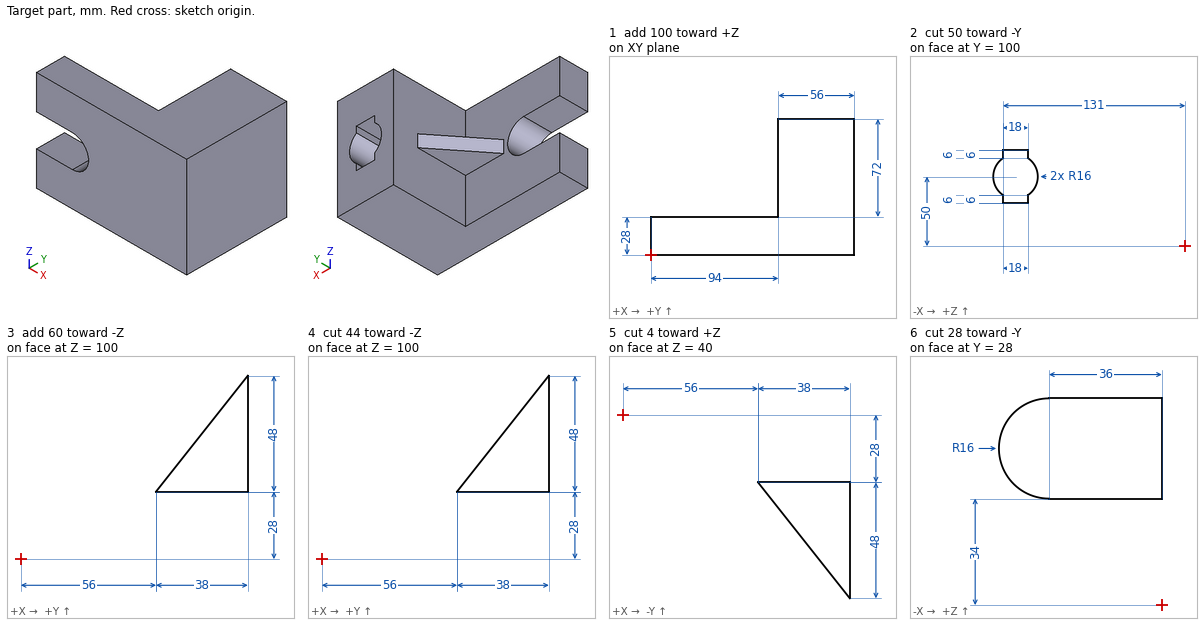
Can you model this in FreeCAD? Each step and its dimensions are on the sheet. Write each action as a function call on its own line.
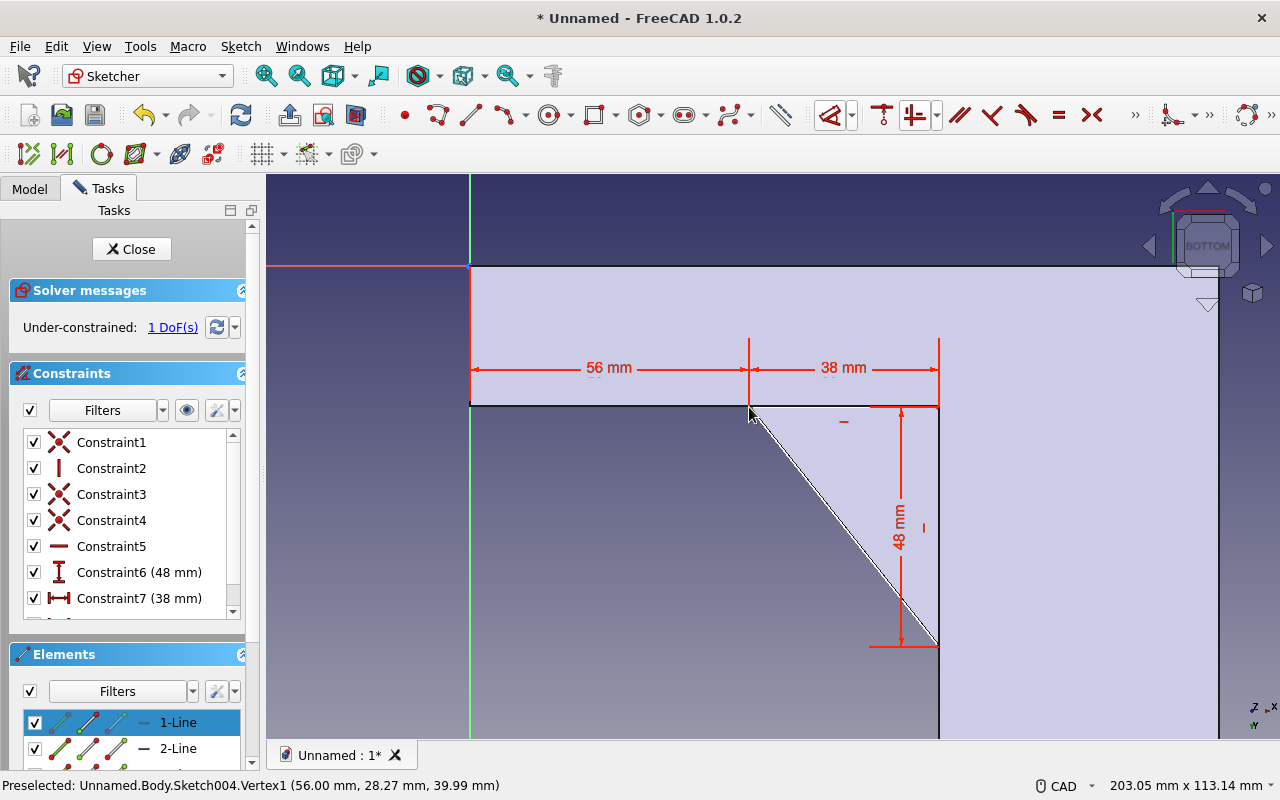
click(852, 116)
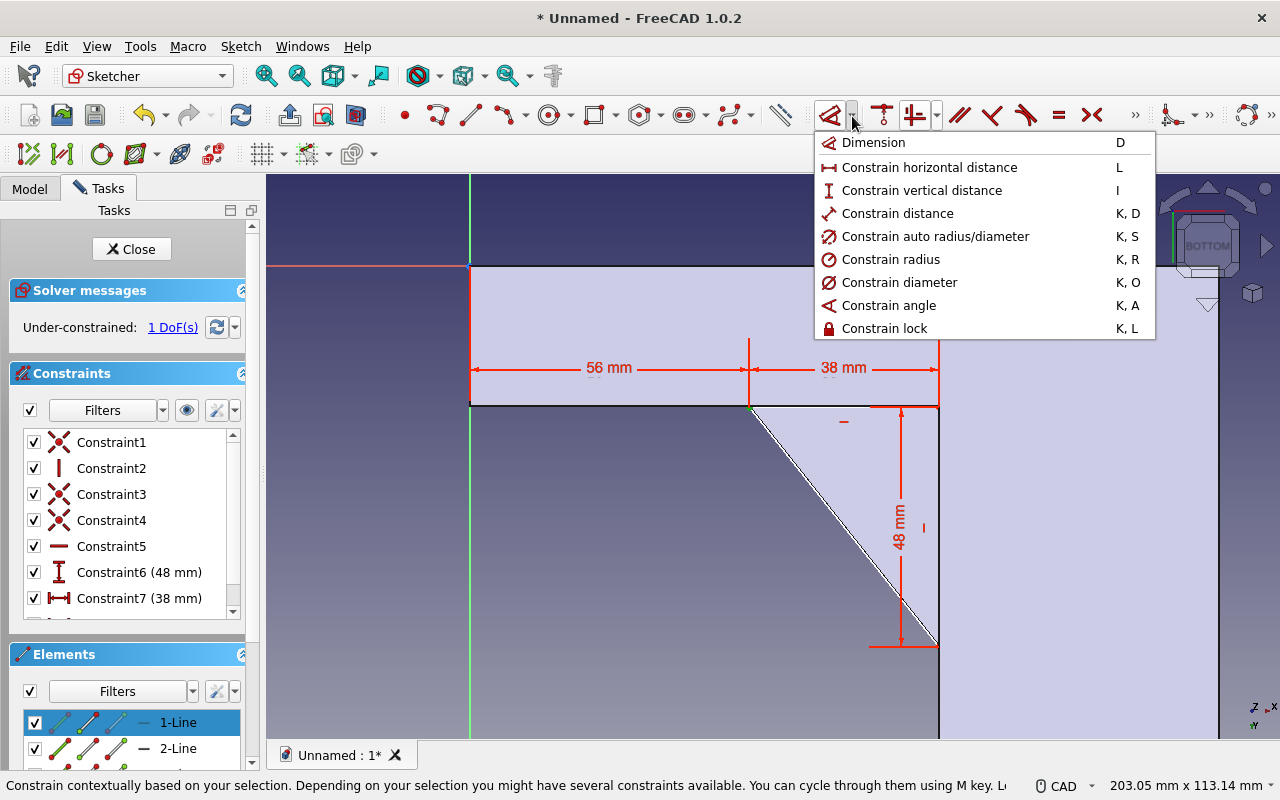
click(985, 190)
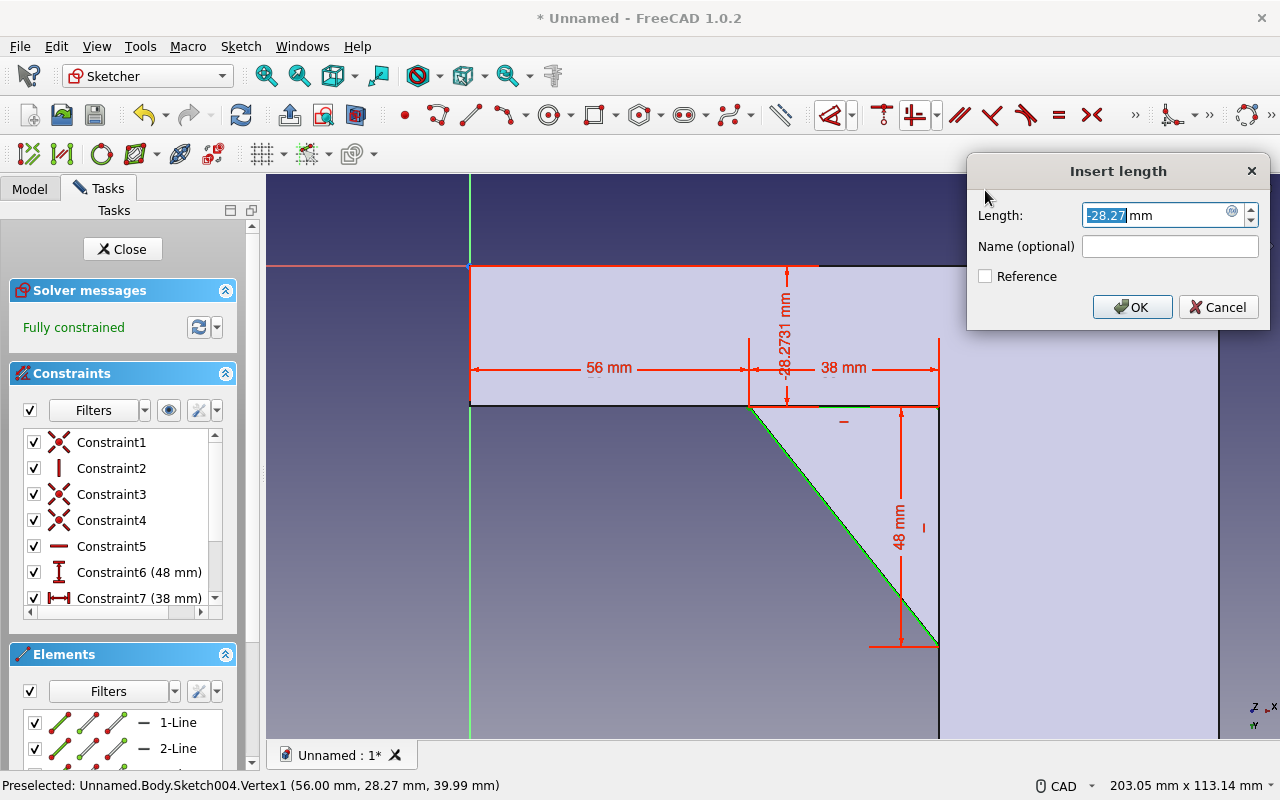
text(-28)
key(Return)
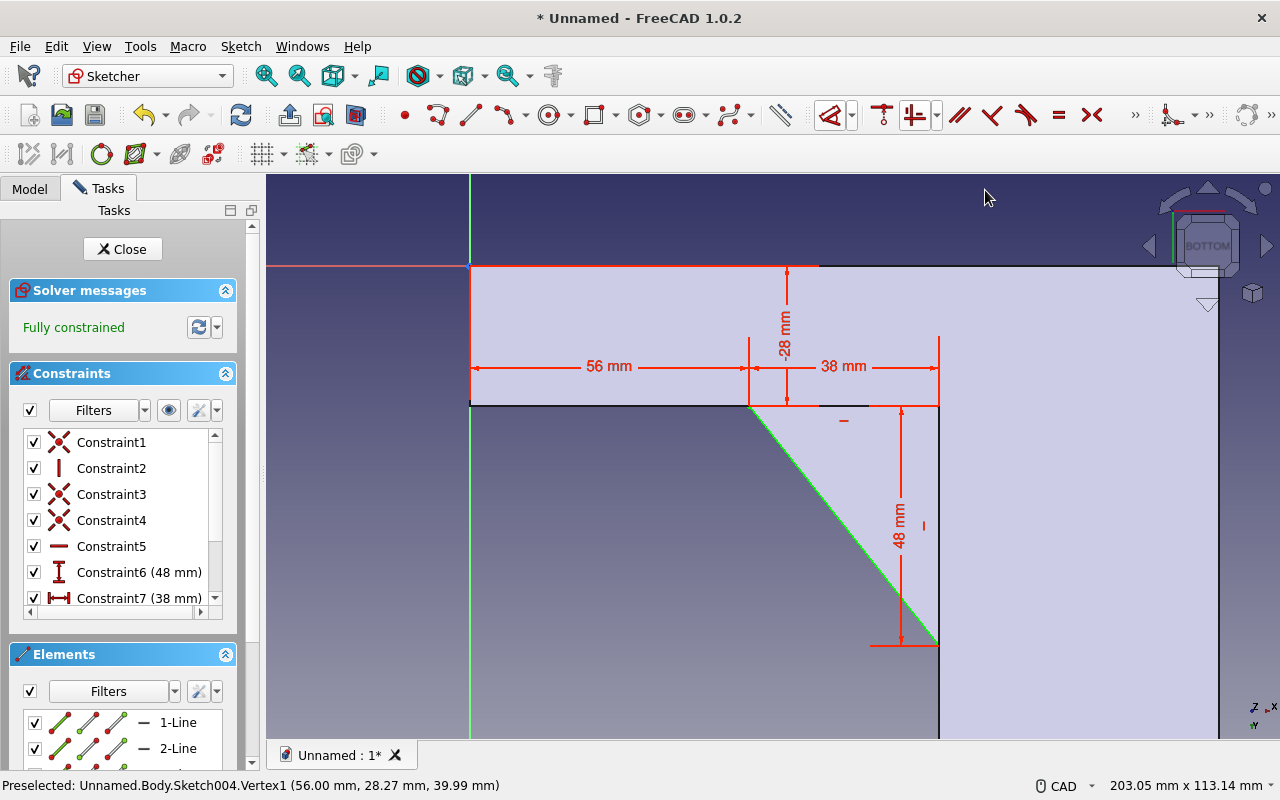
click(123, 249)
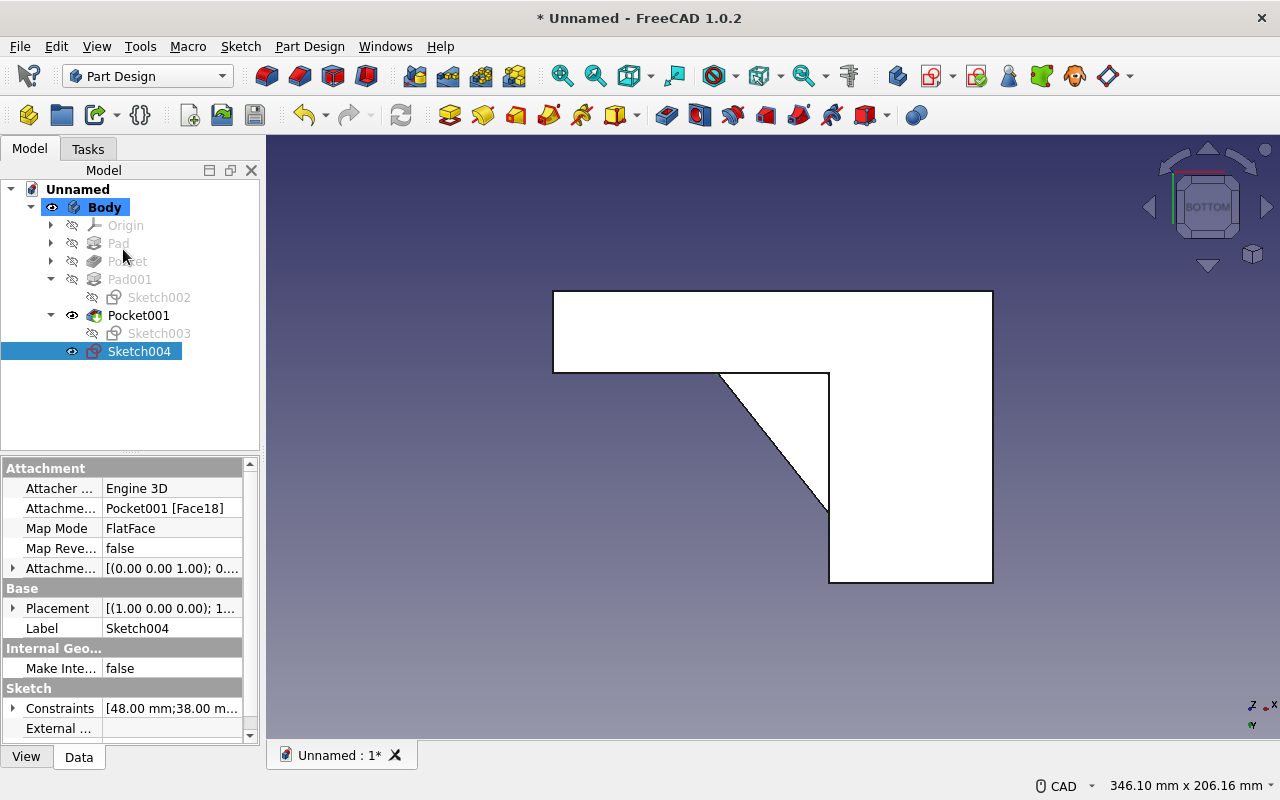
click(667, 116)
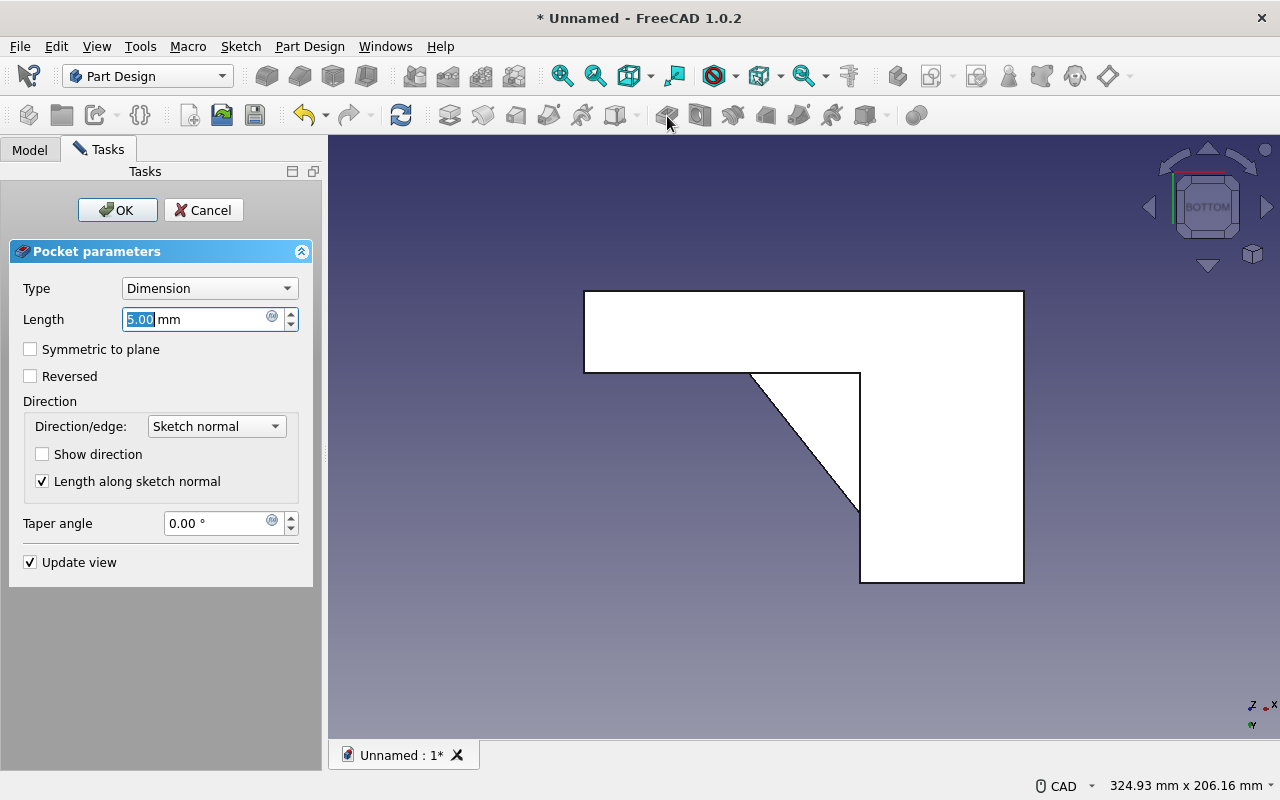
text(4)
key(Tab)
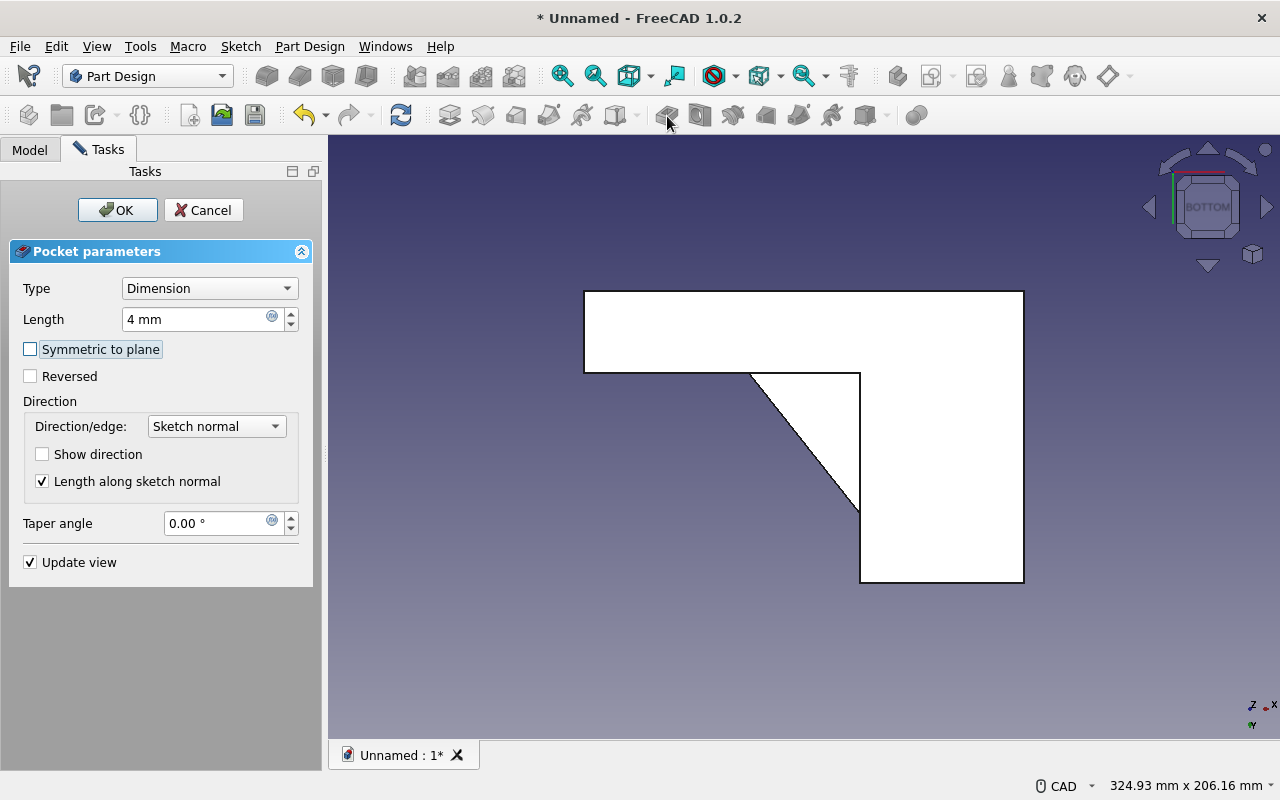
click(118, 210)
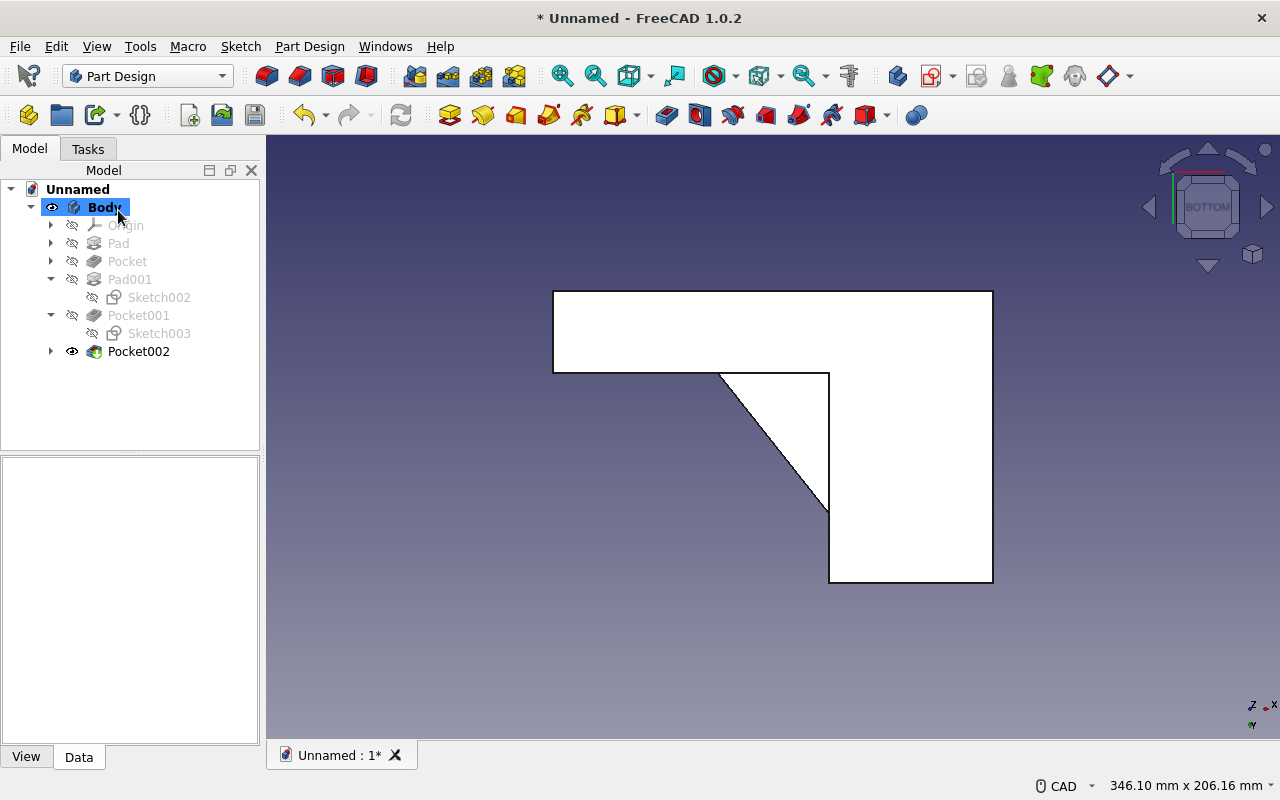
key(4)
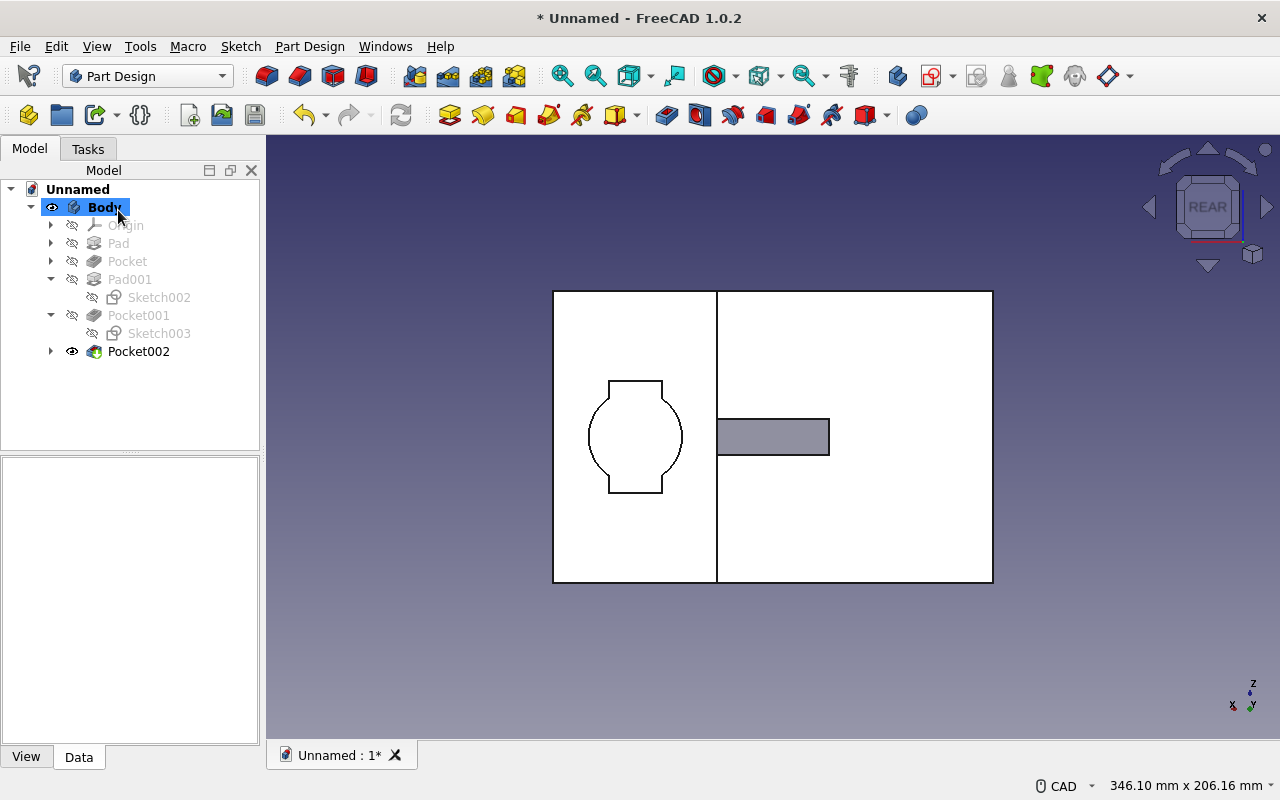
click(894, 394)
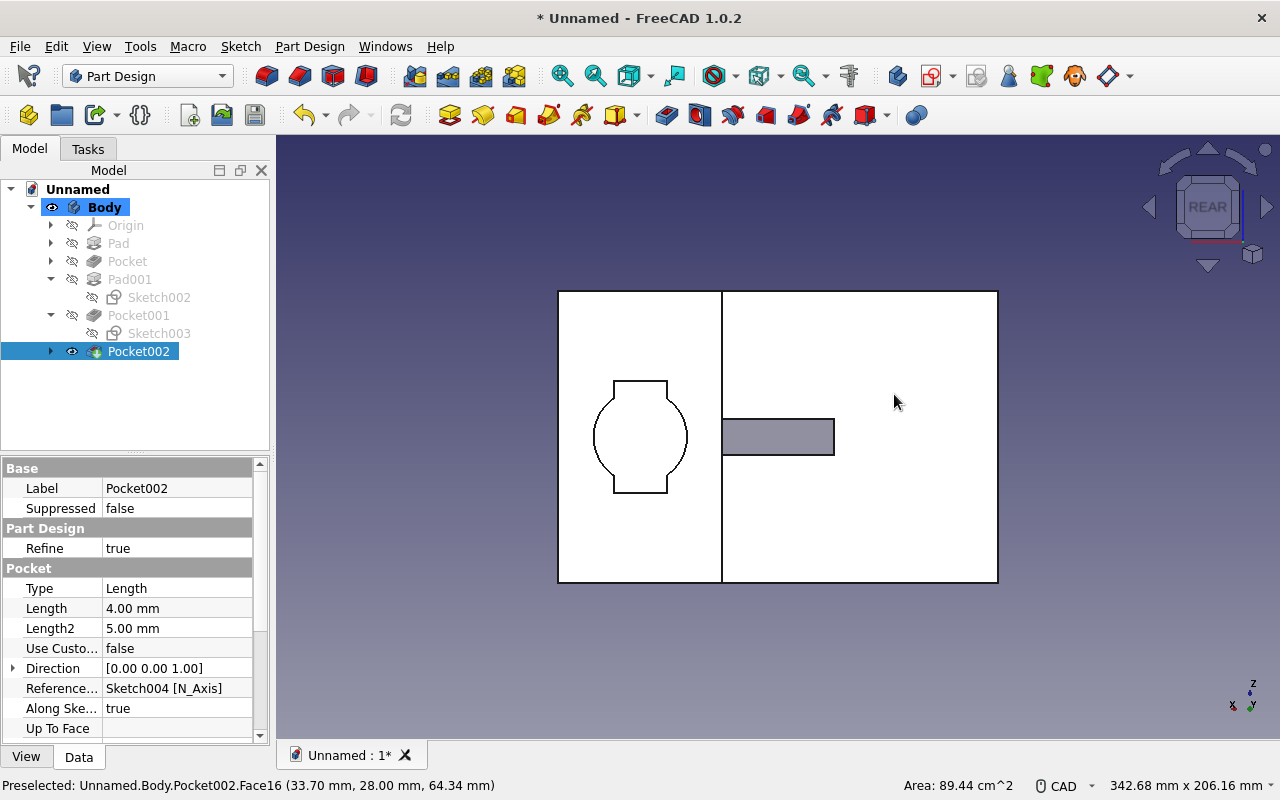
click(930, 76)